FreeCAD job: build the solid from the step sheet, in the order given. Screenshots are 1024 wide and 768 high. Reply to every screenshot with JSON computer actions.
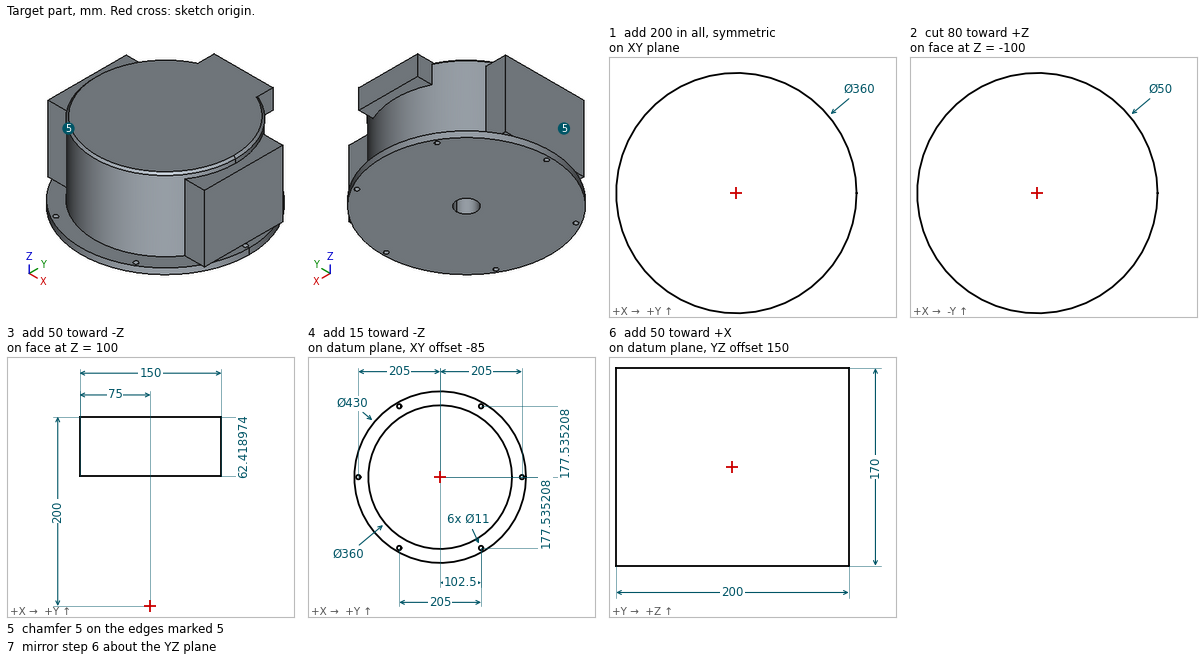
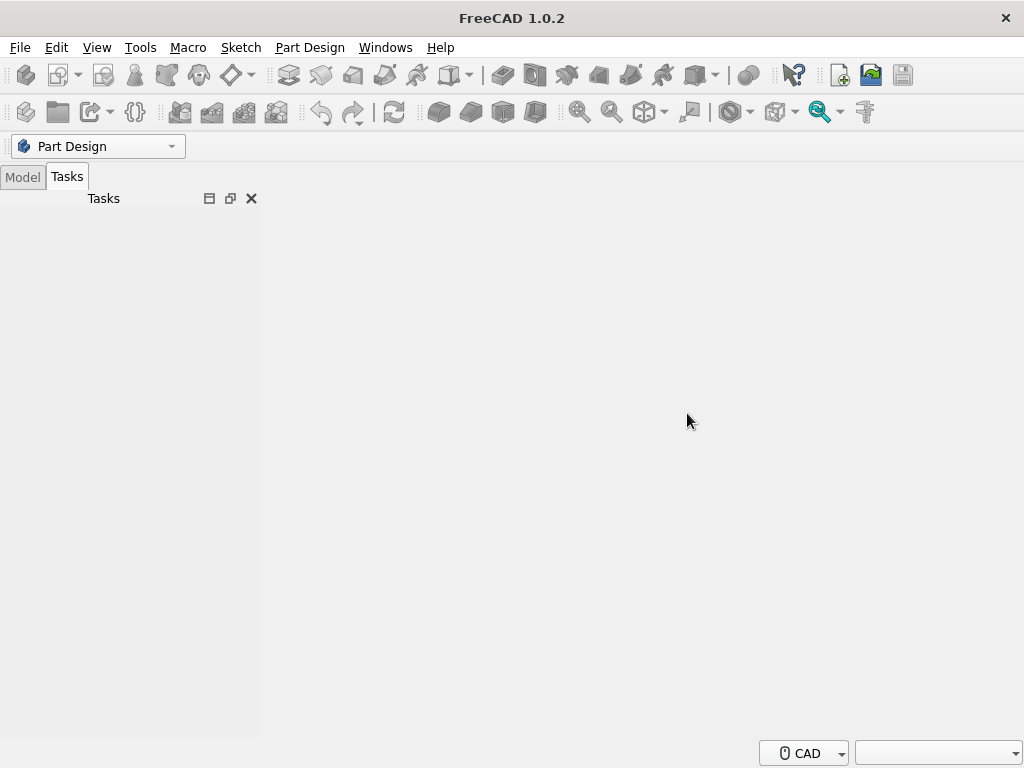
{"action": "left_click", "coordinate": [840, 76]}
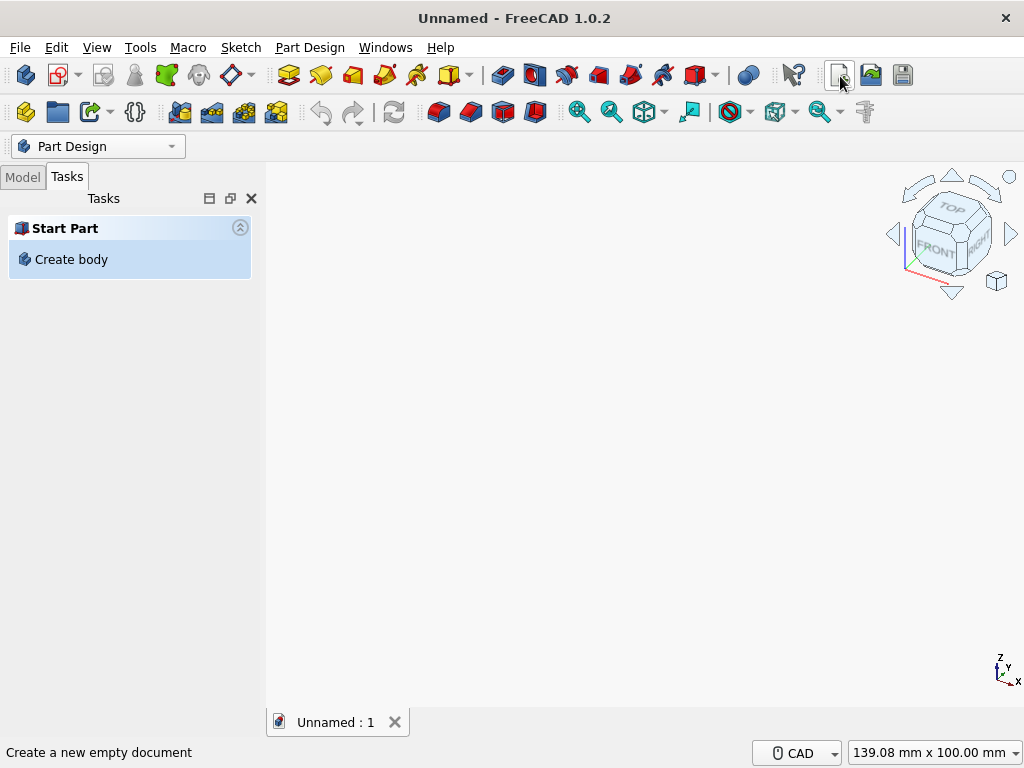
{"action": "left_click", "coordinate": [58, 76]}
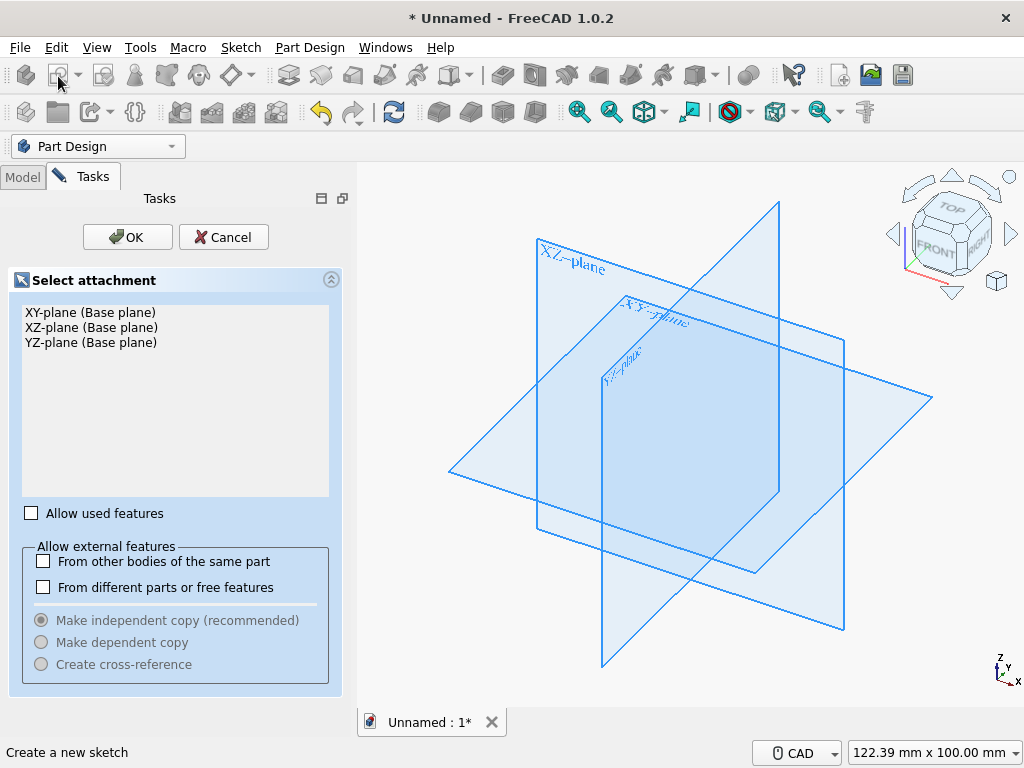
{"action": "left_click", "coordinate": [82, 312]}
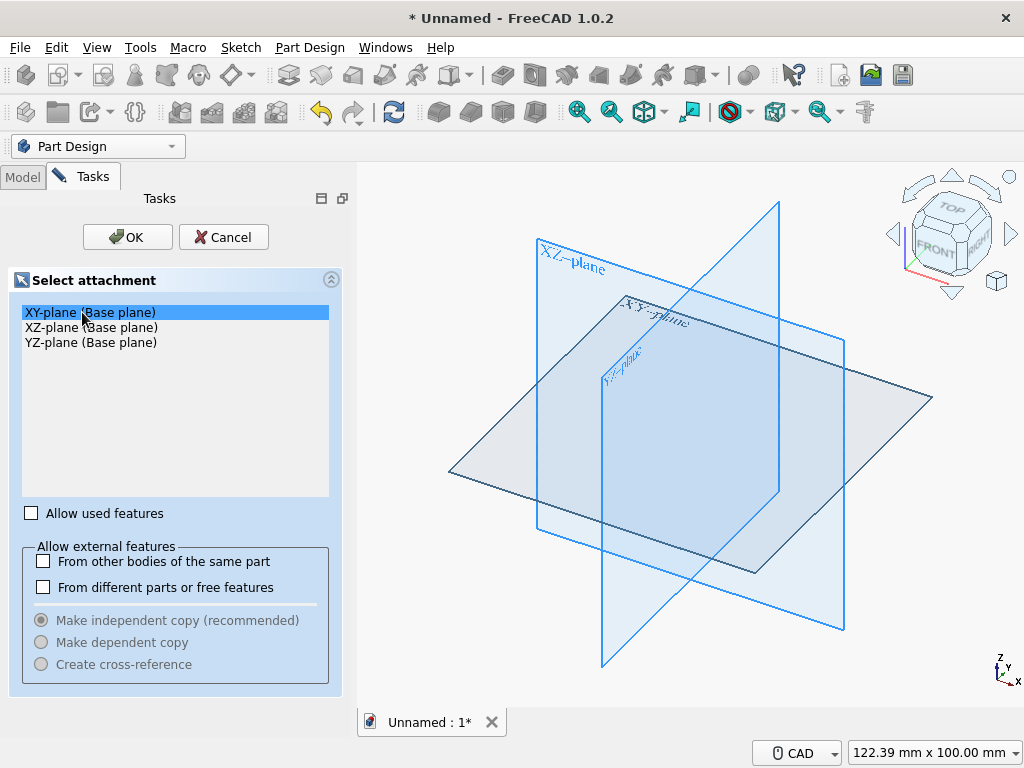
{"action": "left_click", "coordinate": [128, 237]}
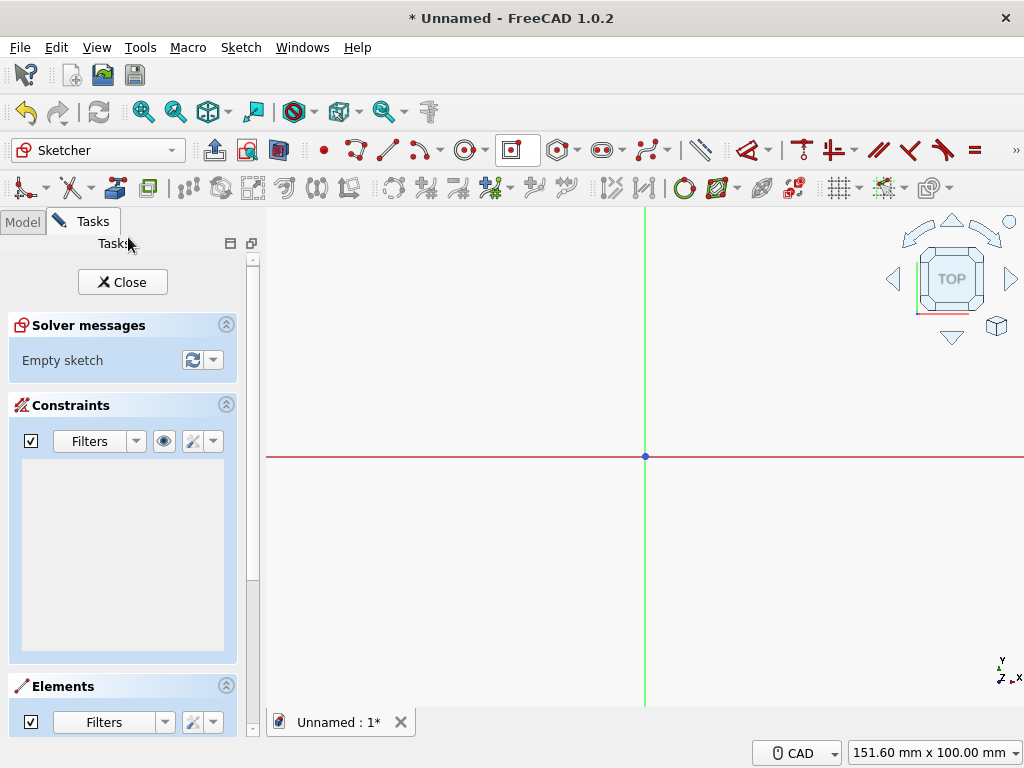
{"action": "scroll", "coordinate": [563, 457], "scroll_direction": "down", "scroll_amount": 9}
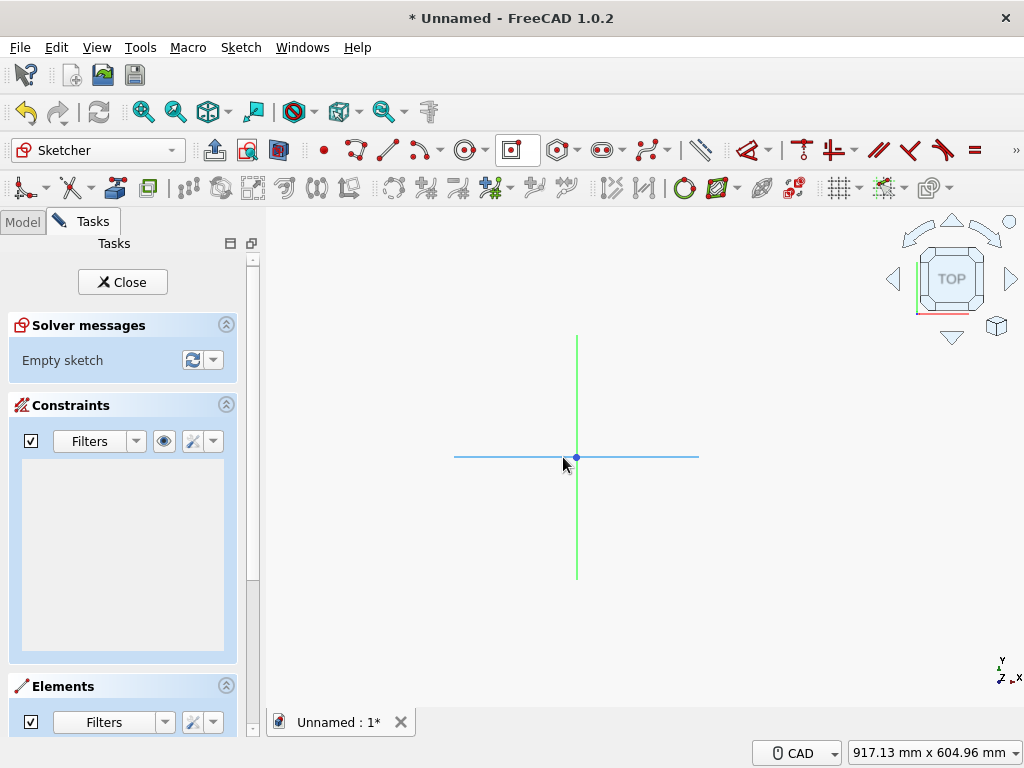
{"action": "left_click", "coordinate": [466, 150]}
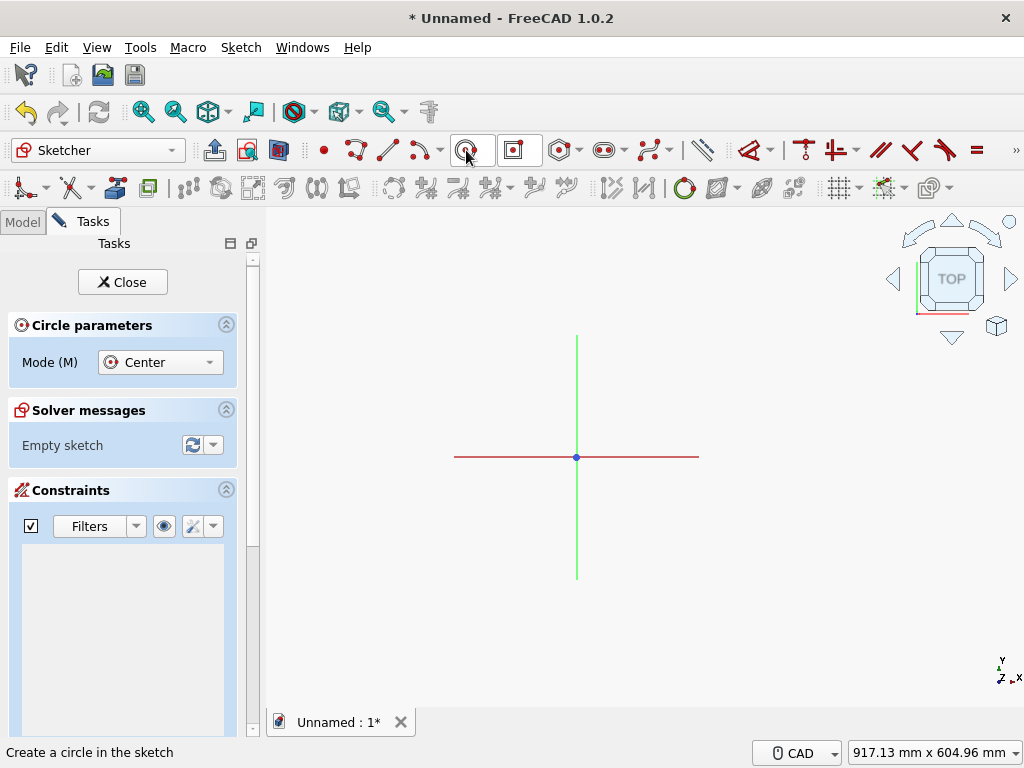
{"action": "left_click", "coordinate": [577, 457]}
{"action": "mouse_move", "coordinate": [682, 352]}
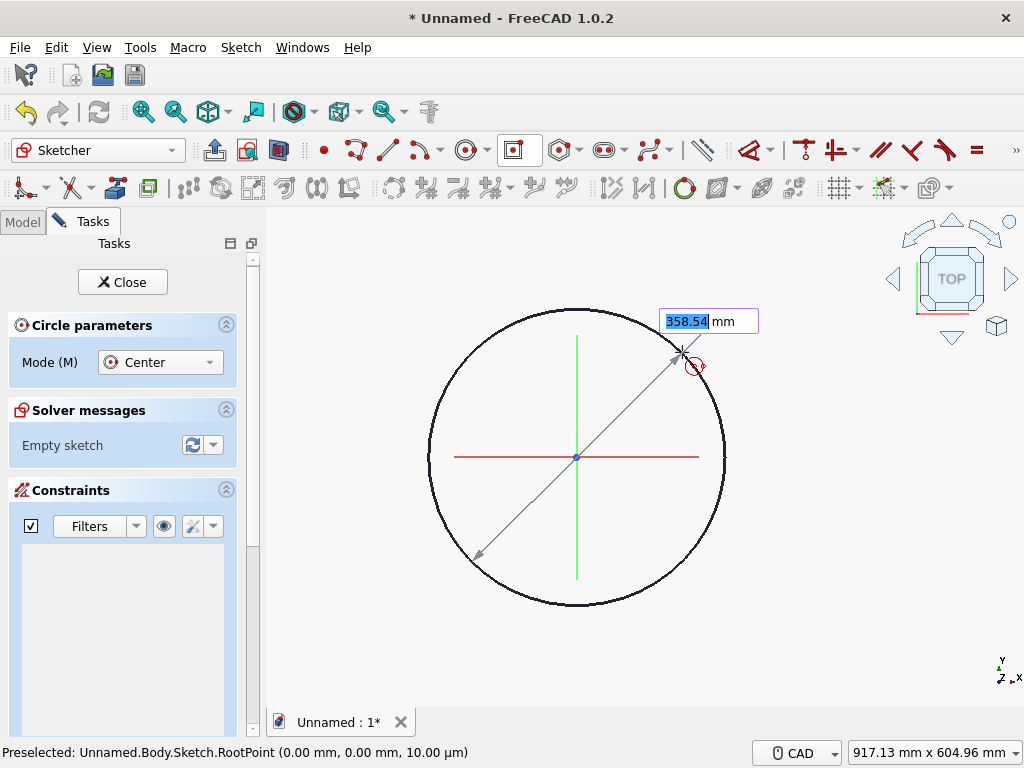
{"action": "type", "text": "360"}
{"action": "key", "text": "Return"}
{"action": "key", "text": "Escape"}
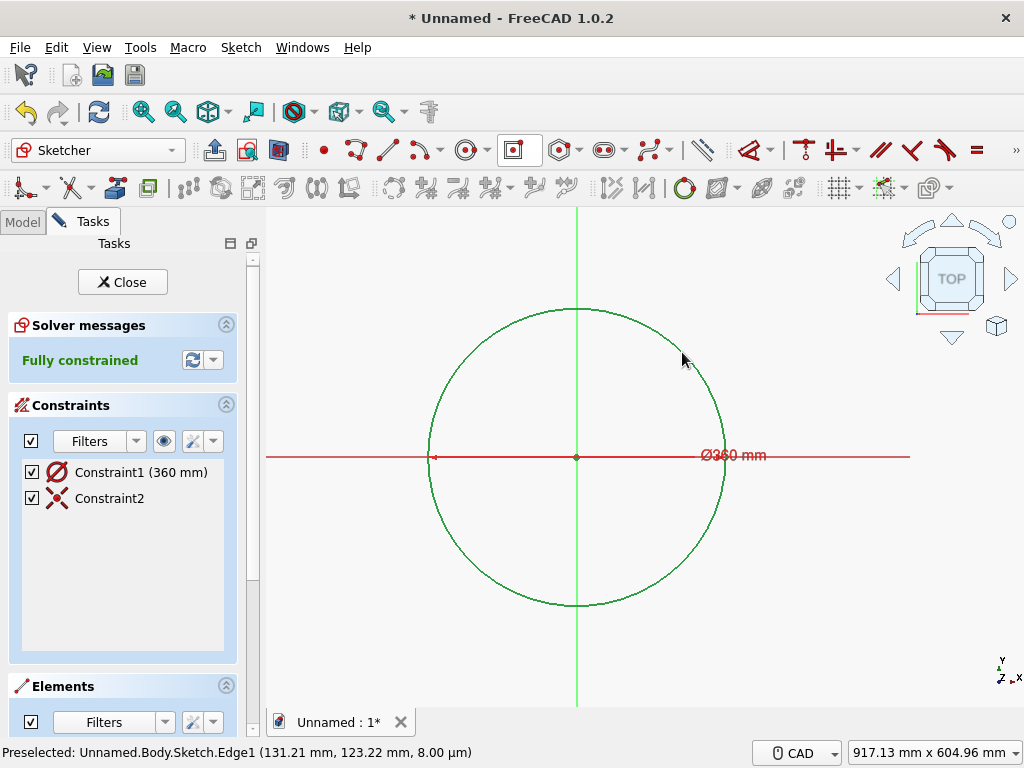
{"action": "left_click", "coordinate": [123, 282]}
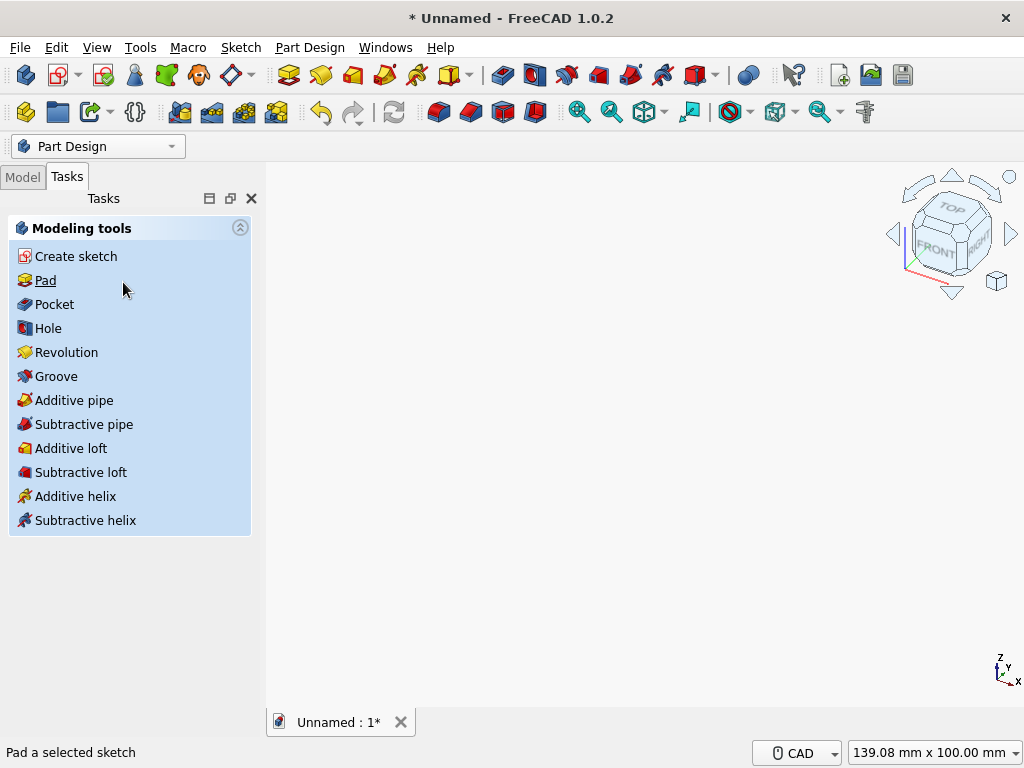
{"action": "left_click", "coordinate": [290, 76]}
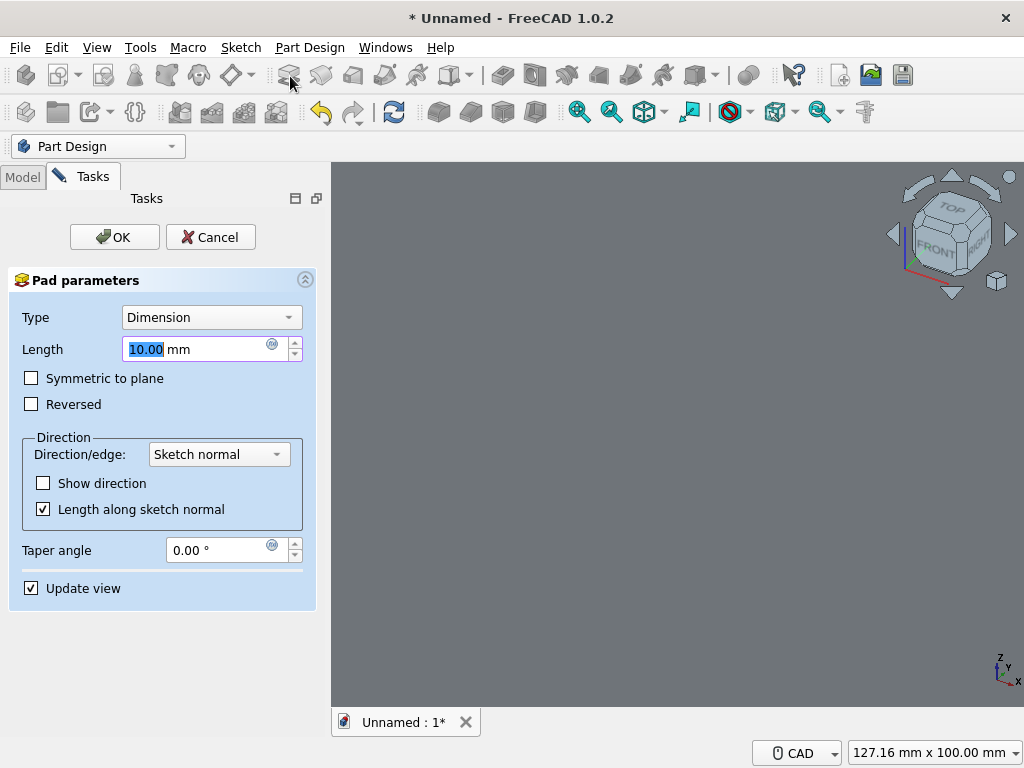
{"action": "type", "text": "200"}
{"action": "key", "text": "Tab"}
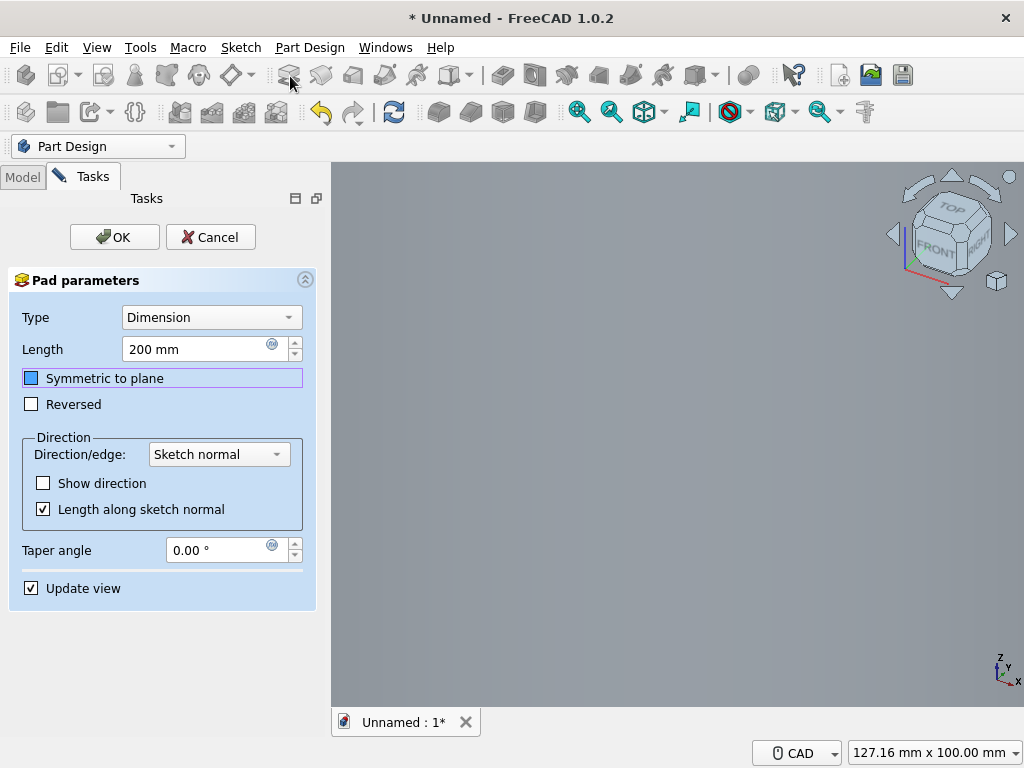
{"action": "left_click", "coordinate": [30, 378]}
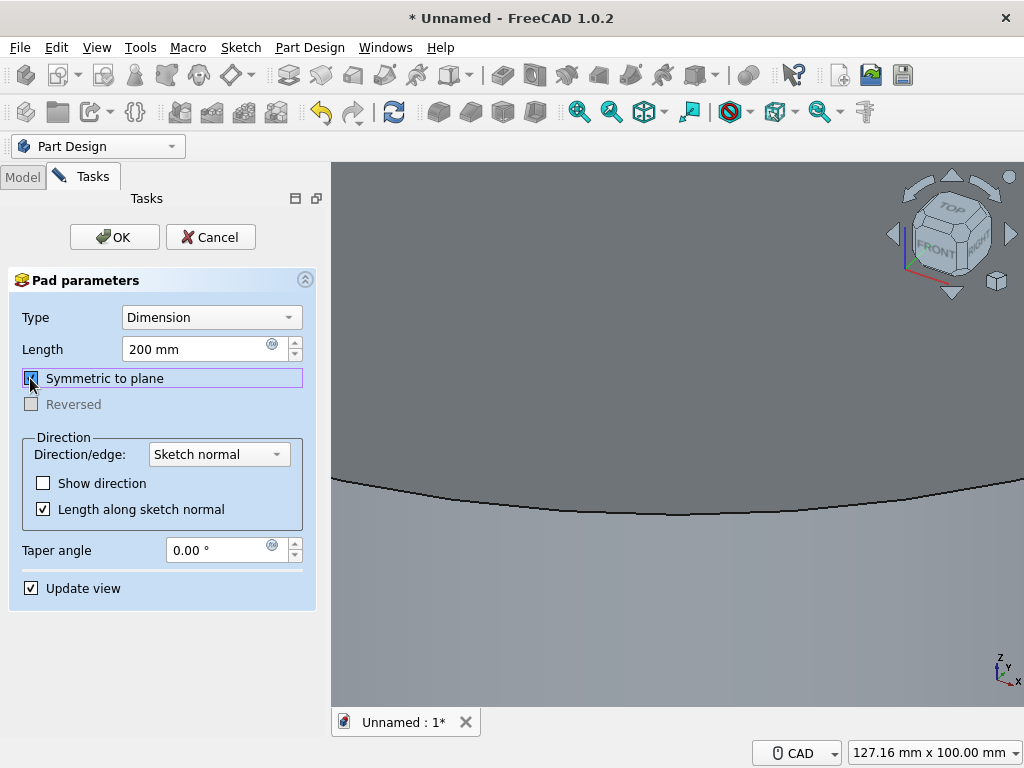
{"action": "left_click", "coordinate": [115, 237]}